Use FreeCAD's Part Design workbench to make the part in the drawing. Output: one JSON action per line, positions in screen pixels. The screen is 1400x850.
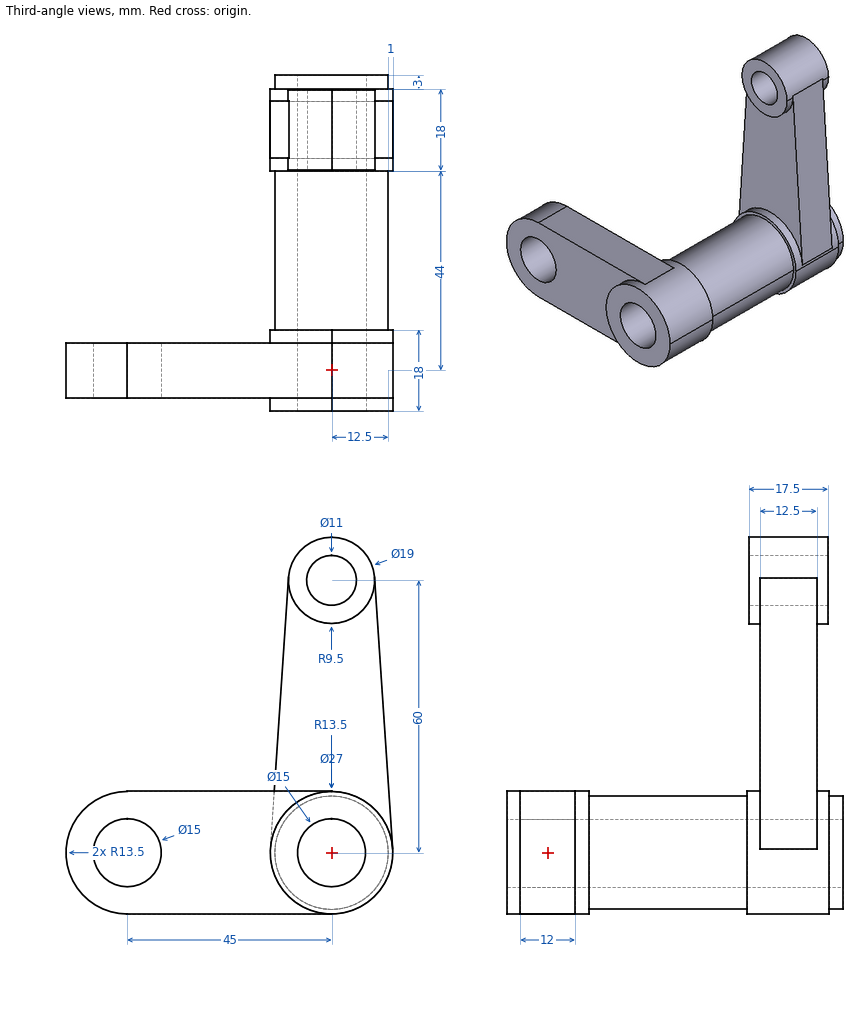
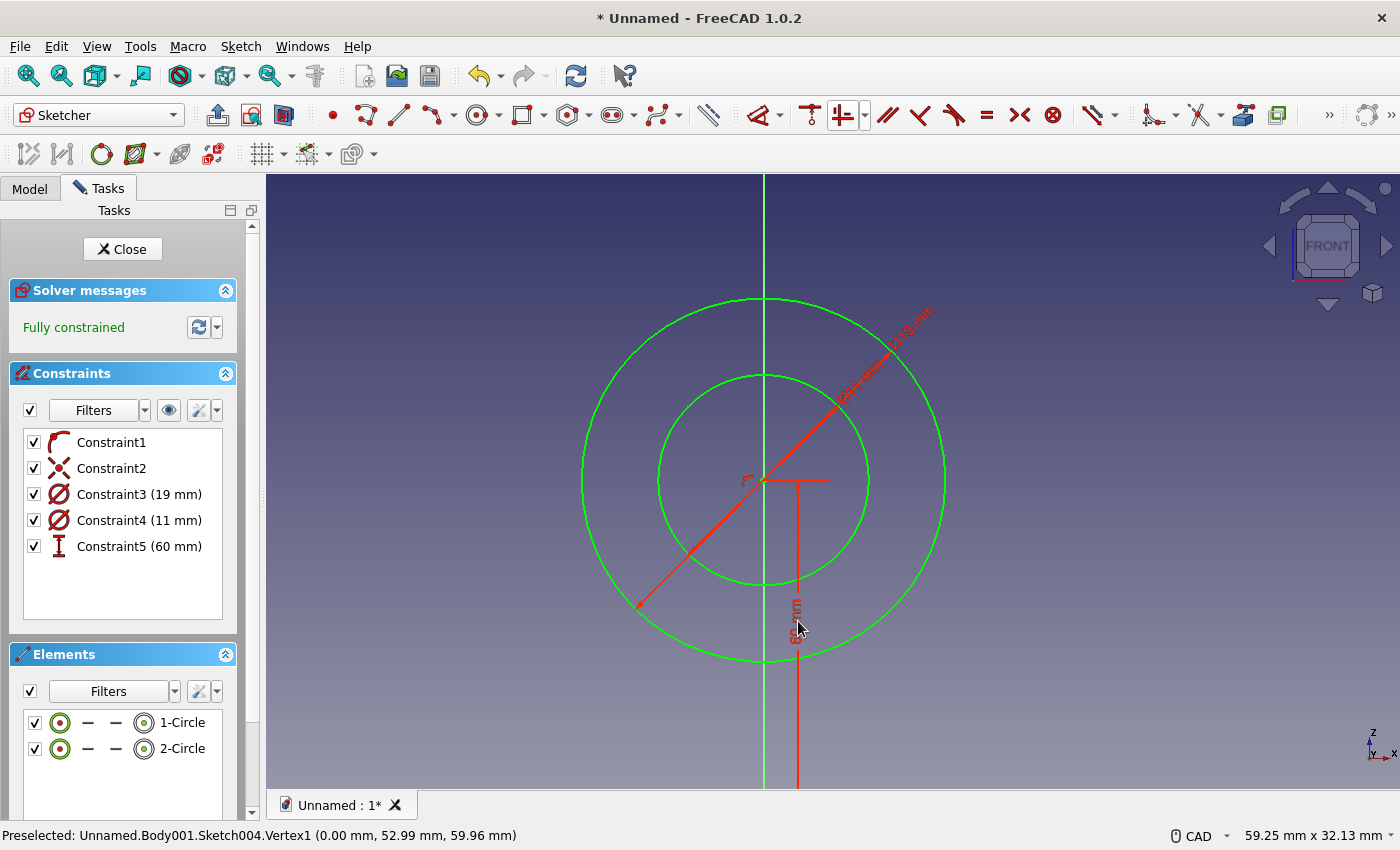
{"action": "left_click", "coordinate": [123, 249]}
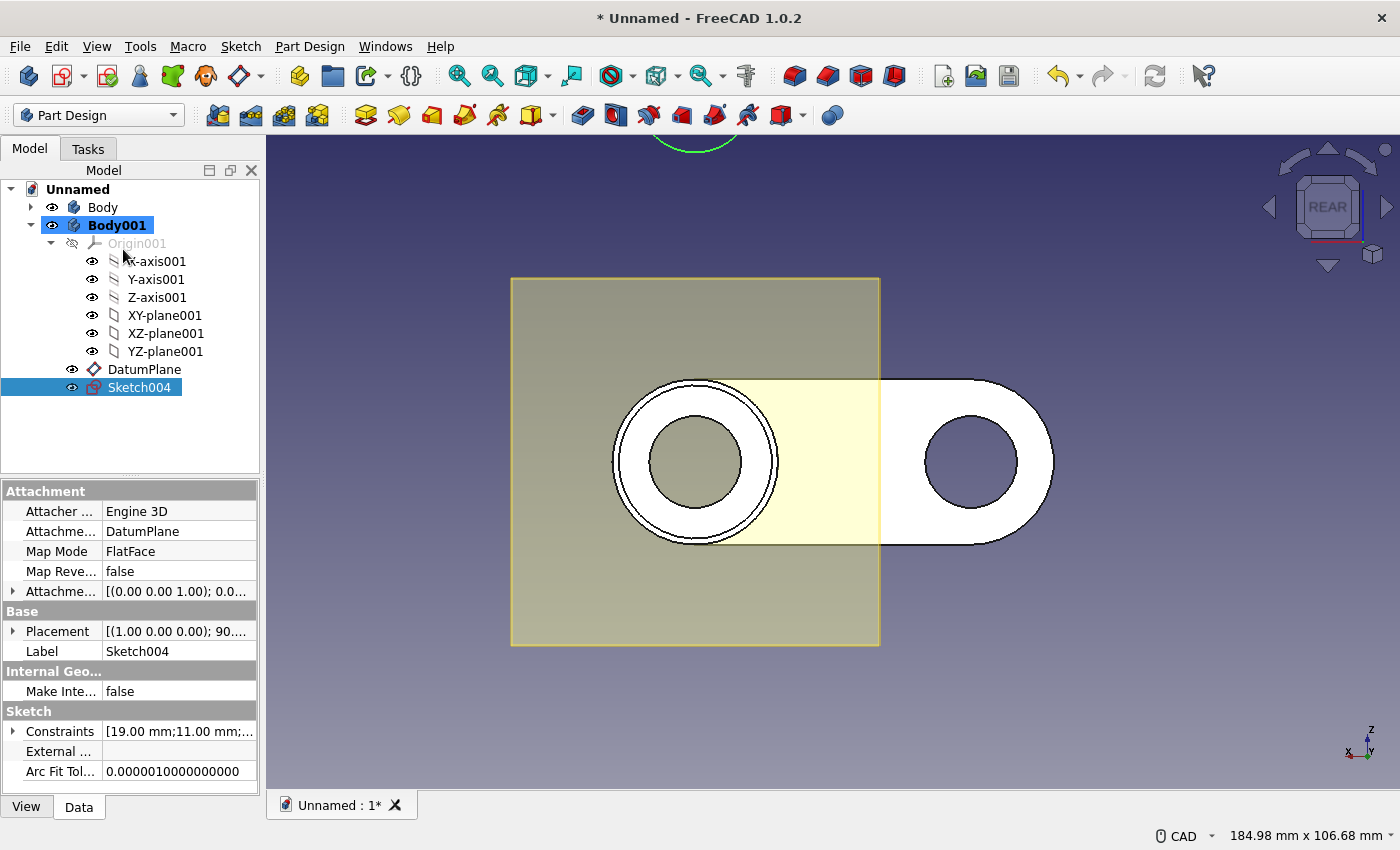
{"action": "left_click", "coordinate": [366, 116]}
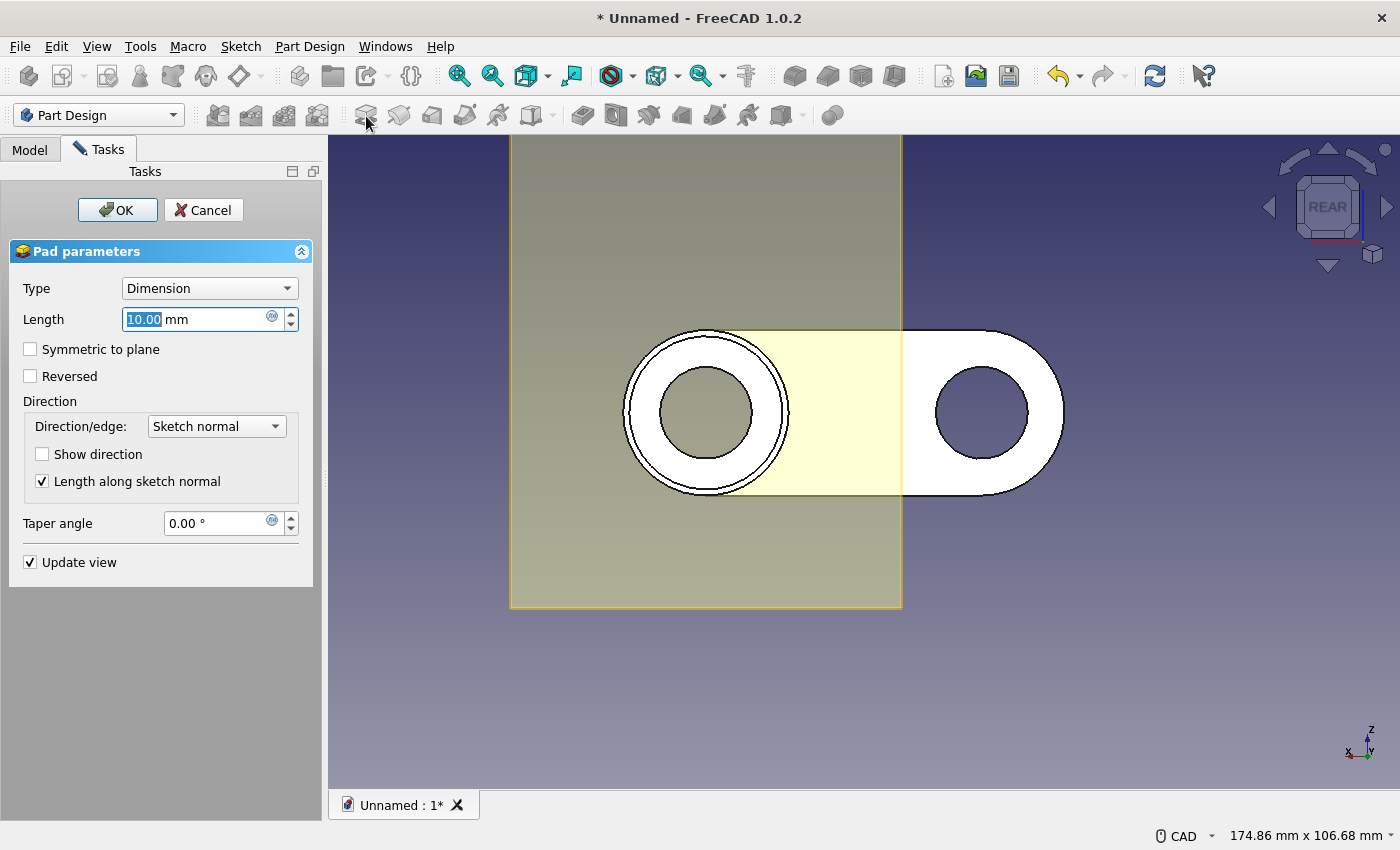
{"action": "type", "text": "17.5"}
{"action": "key", "text": "Tab"}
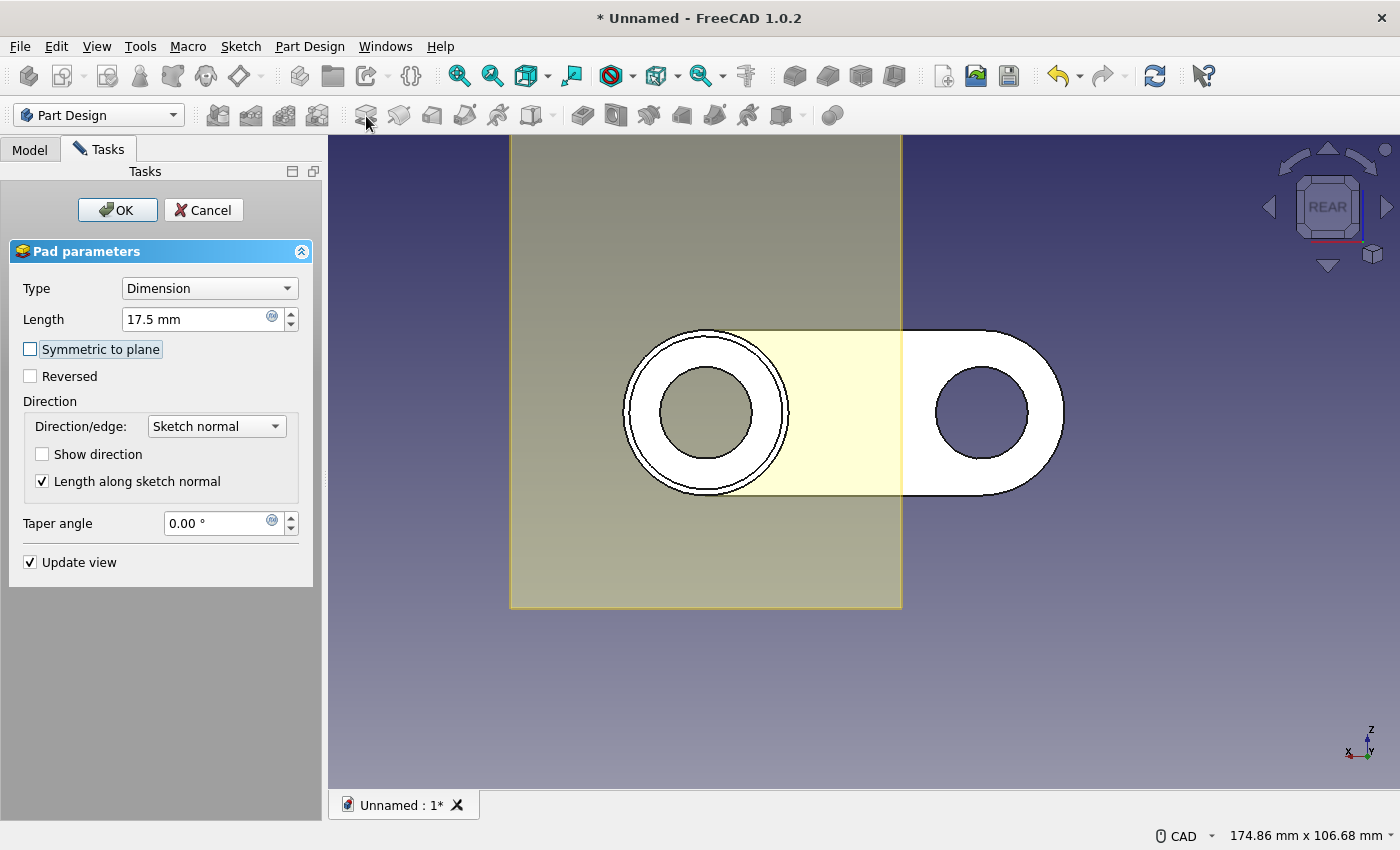
{"action": "left_click", "coordinate": [31, 349]}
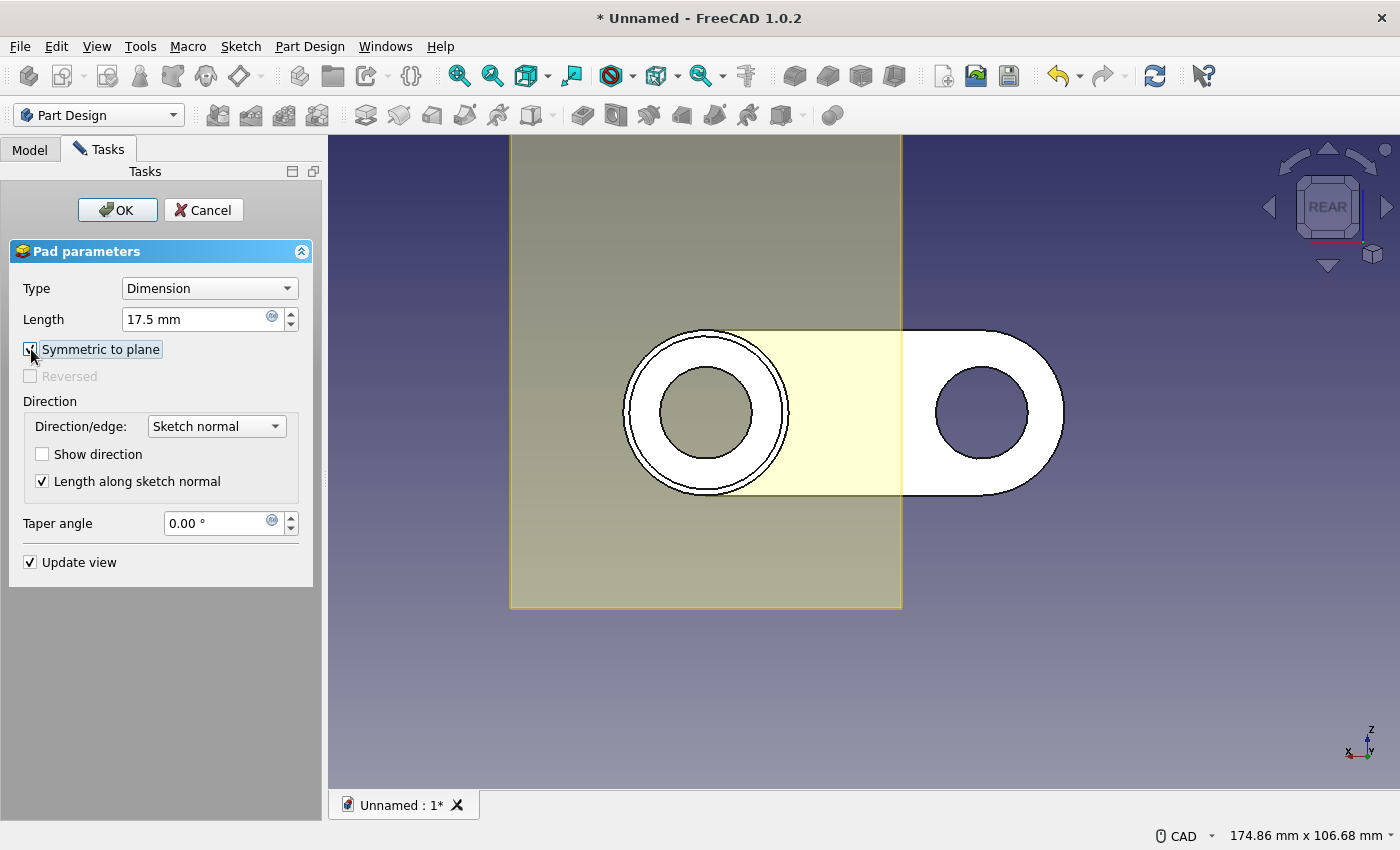
{"action": "left_click", "coordinate": [118, 210]}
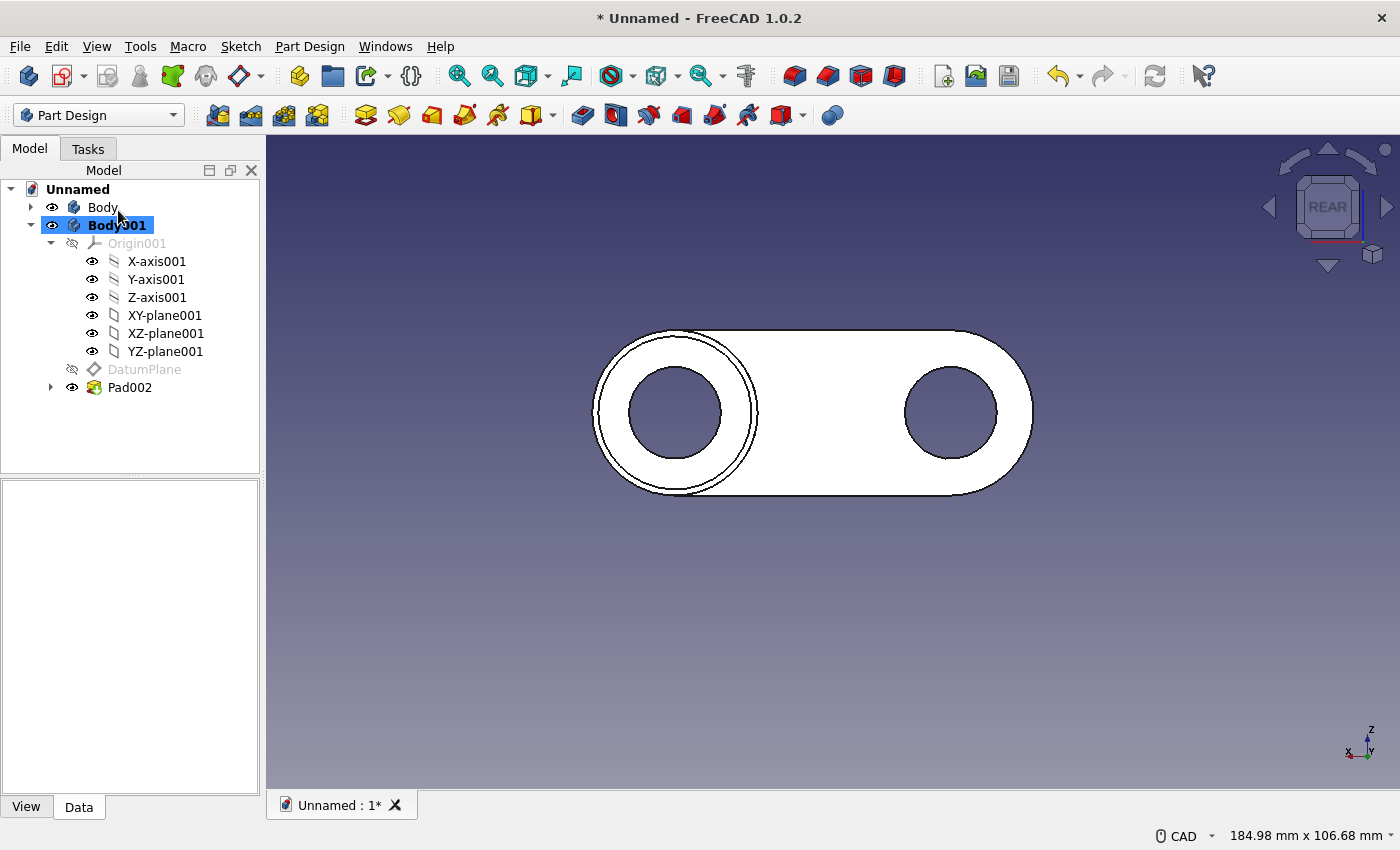
{"action": "left_click", "coordinate": [460, 76]}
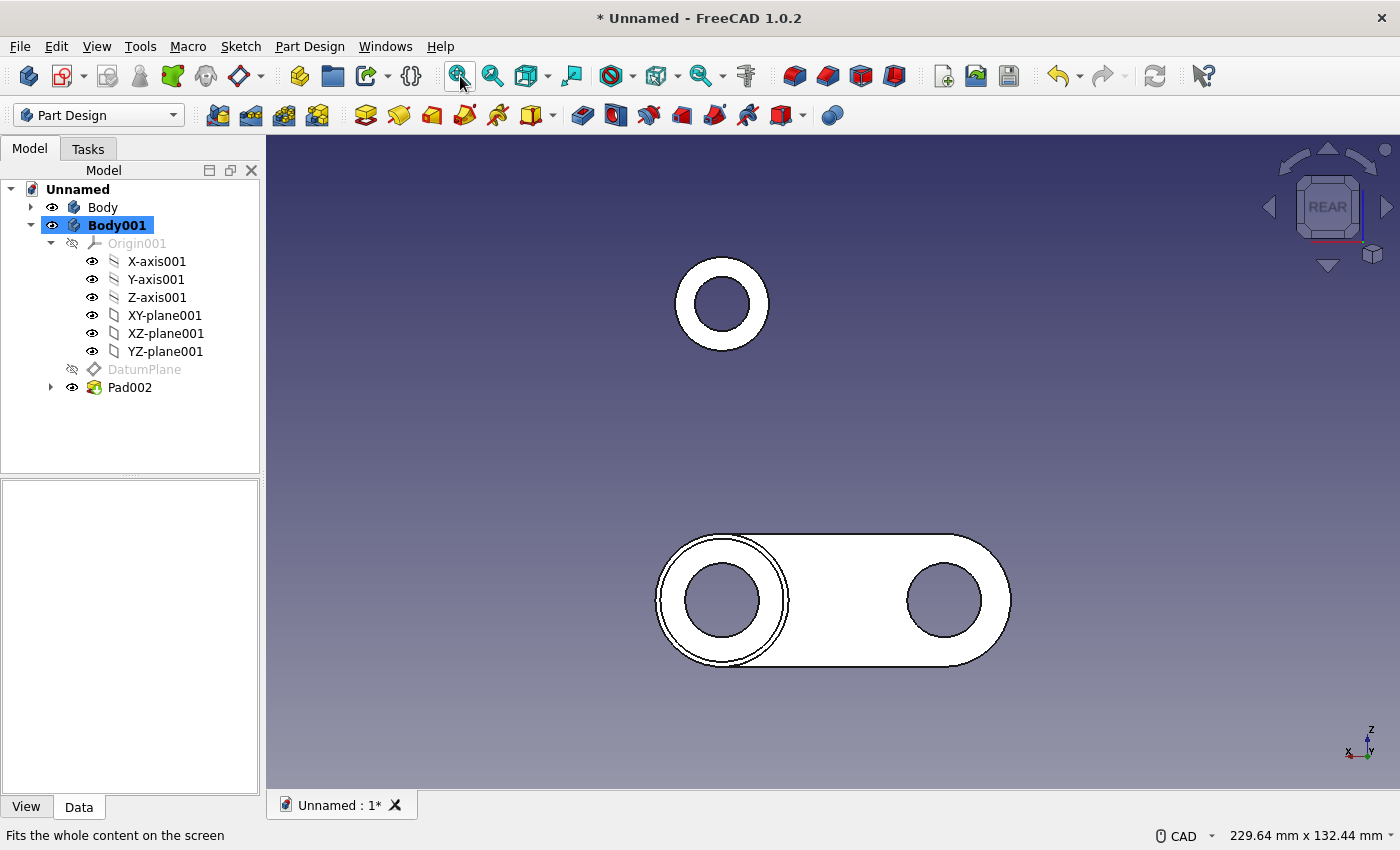
{"action": "double_click", "coordinate": [97, 207]}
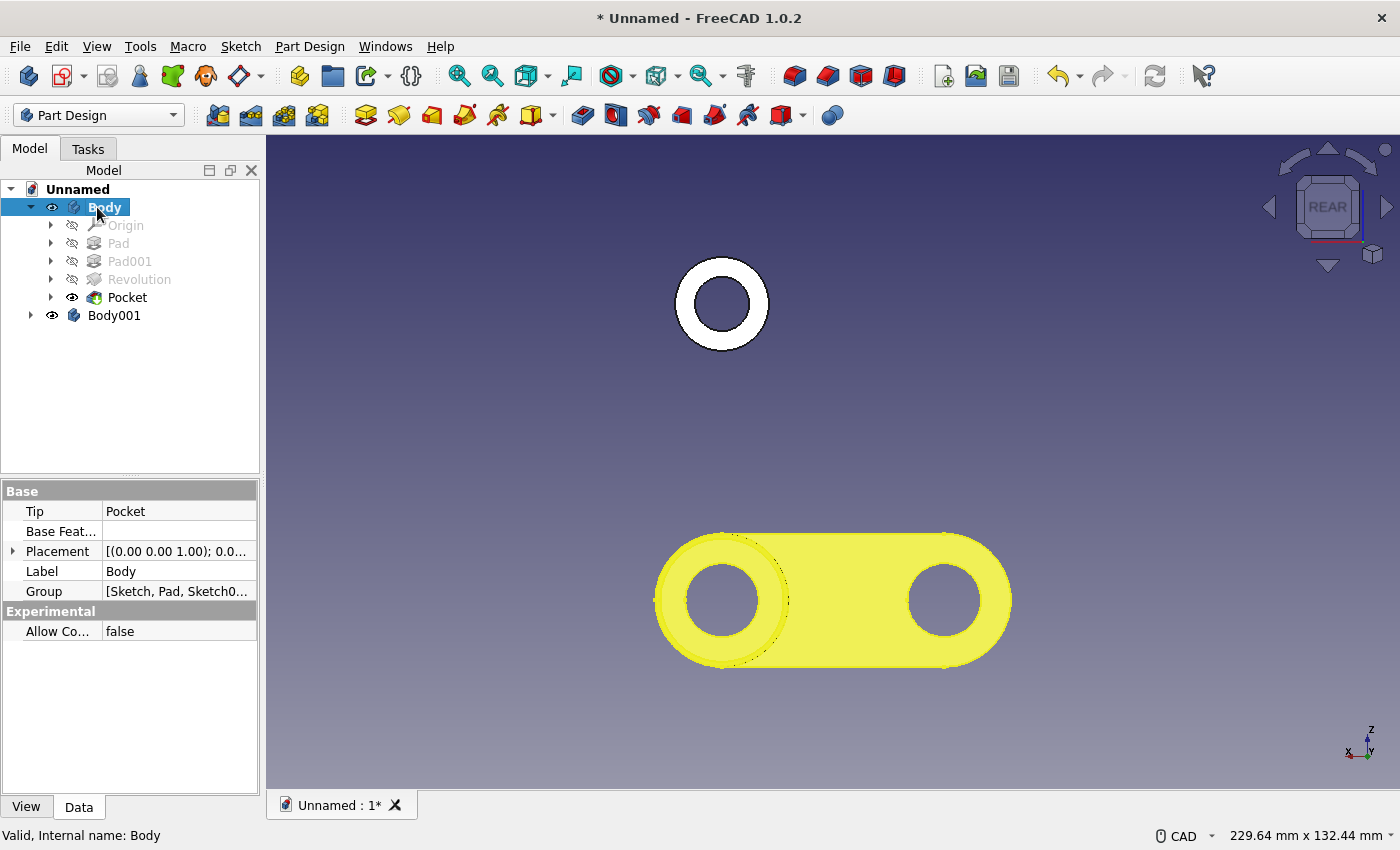
{"action": "left_click", "coordinate": [97, 207]}